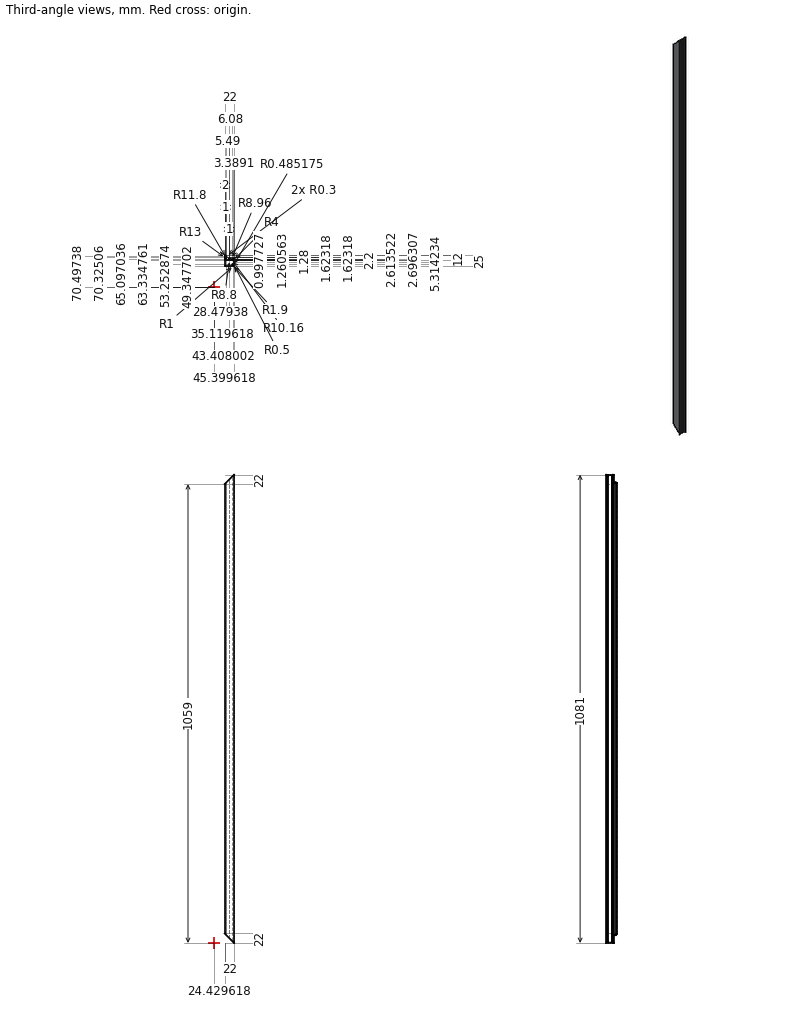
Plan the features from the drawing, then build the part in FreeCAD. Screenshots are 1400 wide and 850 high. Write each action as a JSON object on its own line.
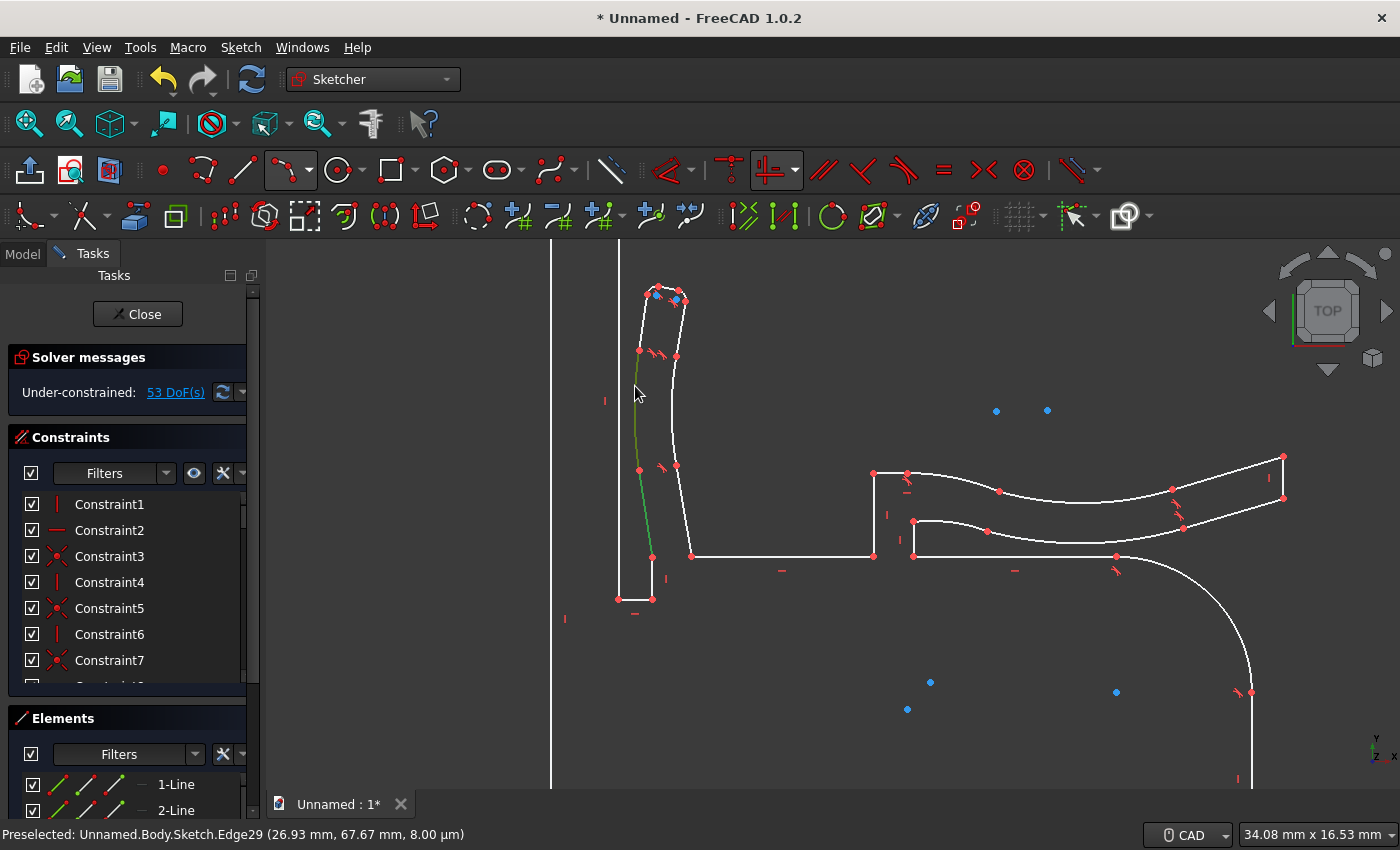
{"action": "left_click", "coordinate": [904, 170]}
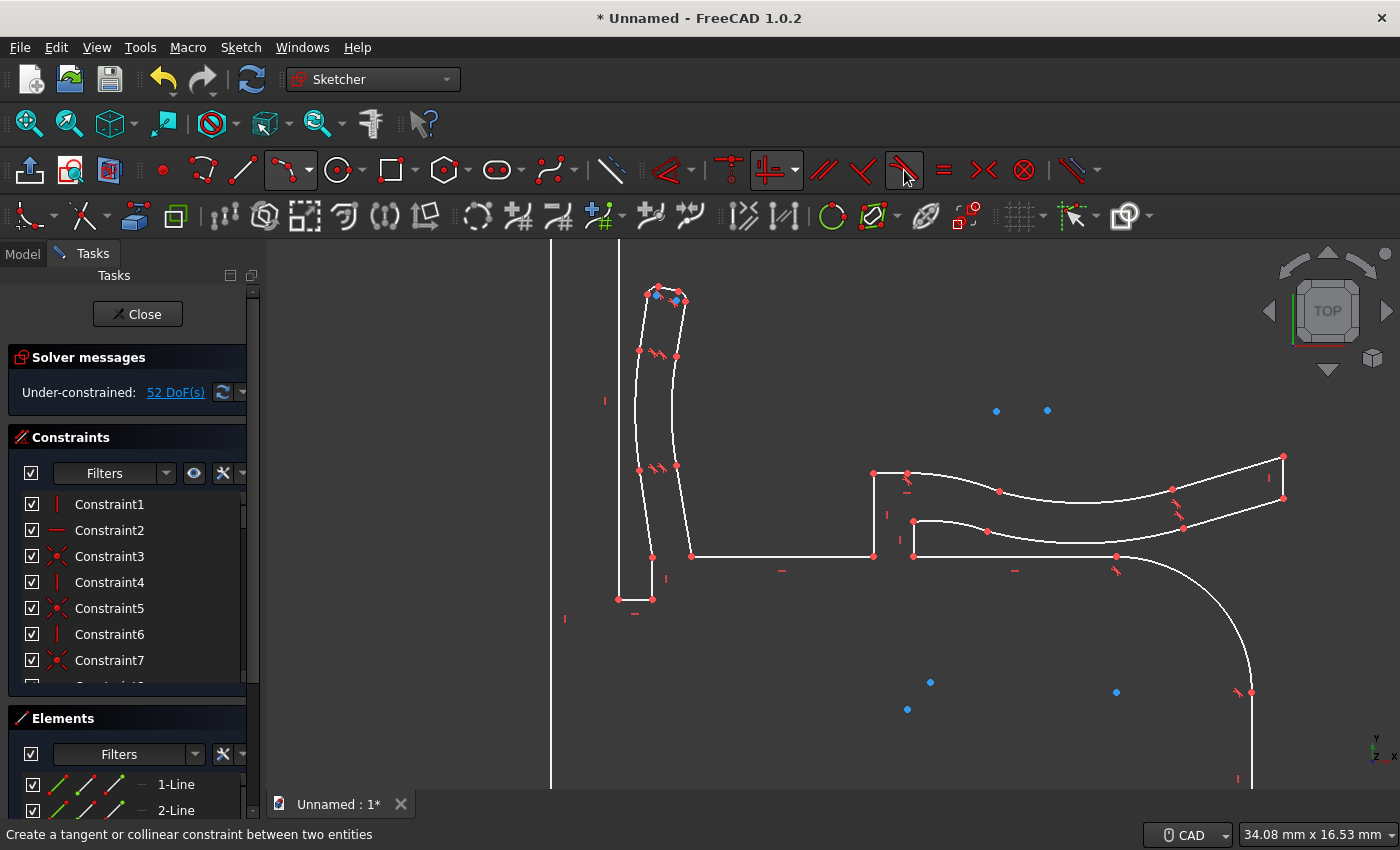
{"action": "scroll", "coordinate": [639, 431], "scroll_direction": "down", "scroll_amount": 4}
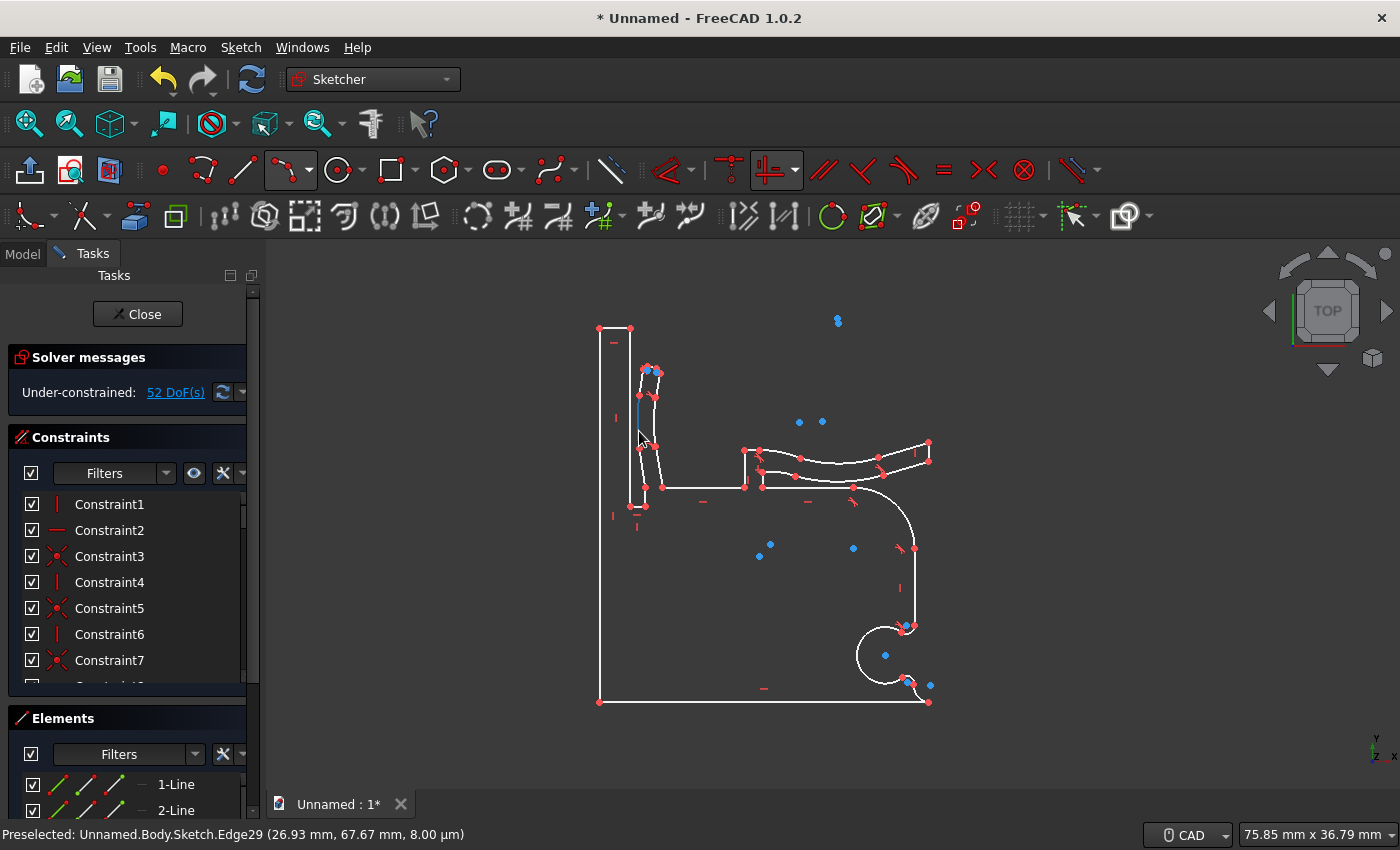
{"action": "left_click", "coordinate": [698, 702]}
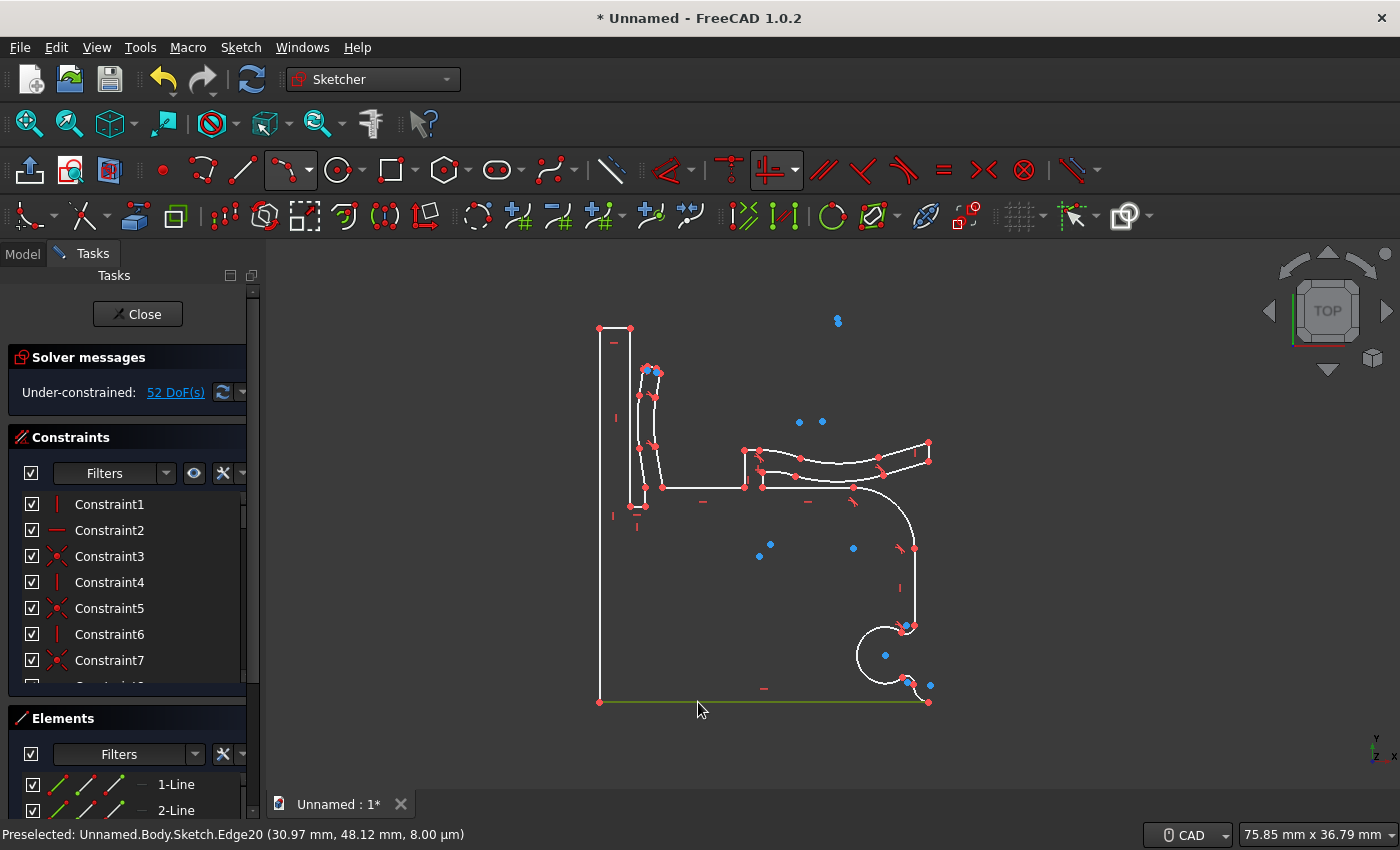
{"action": "scroll", "coordinate": [915, 692], "scroll_direction": "up", "scroll_amount": 3}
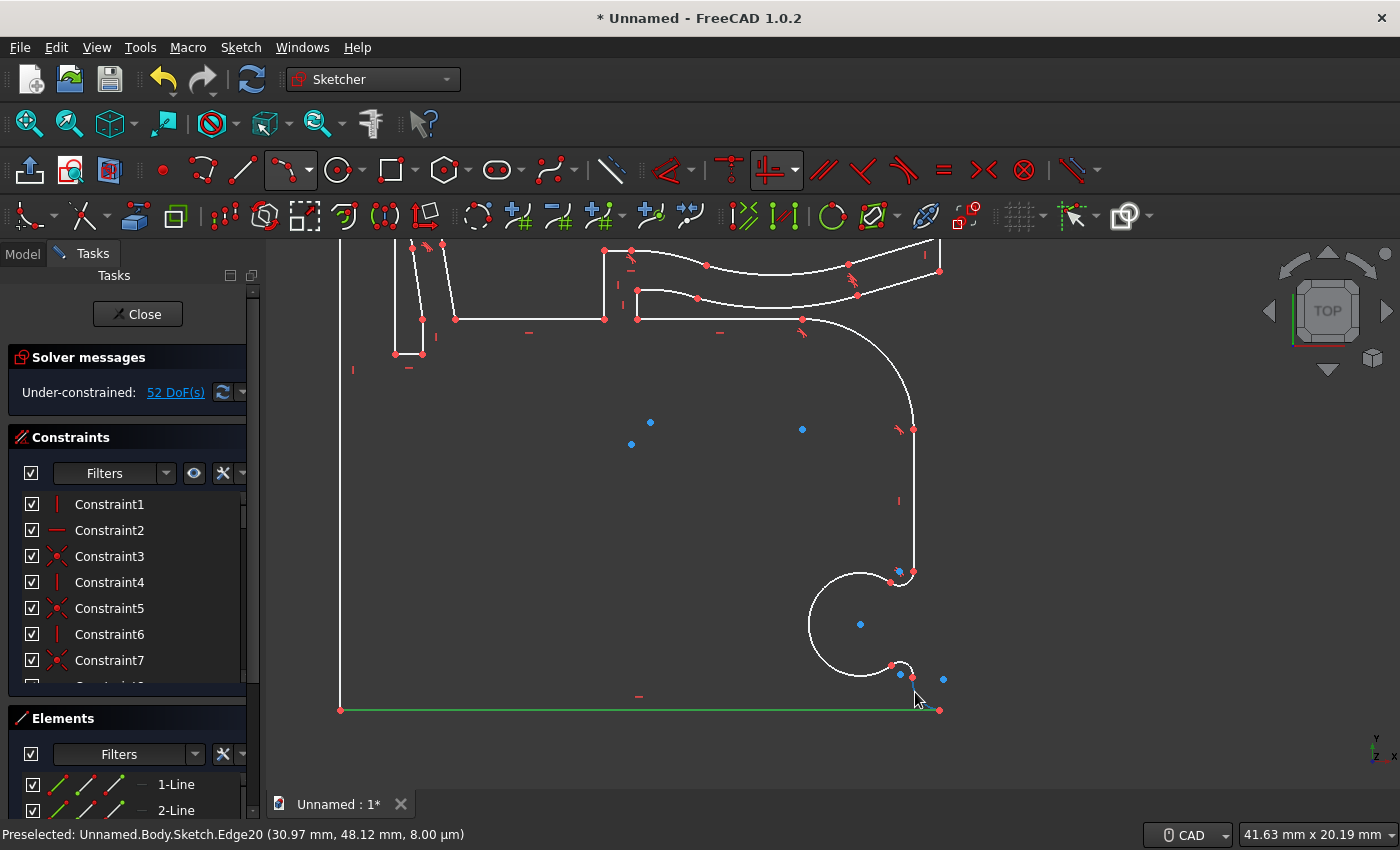
{"action": "left_click", "coordinate": [915, 692]}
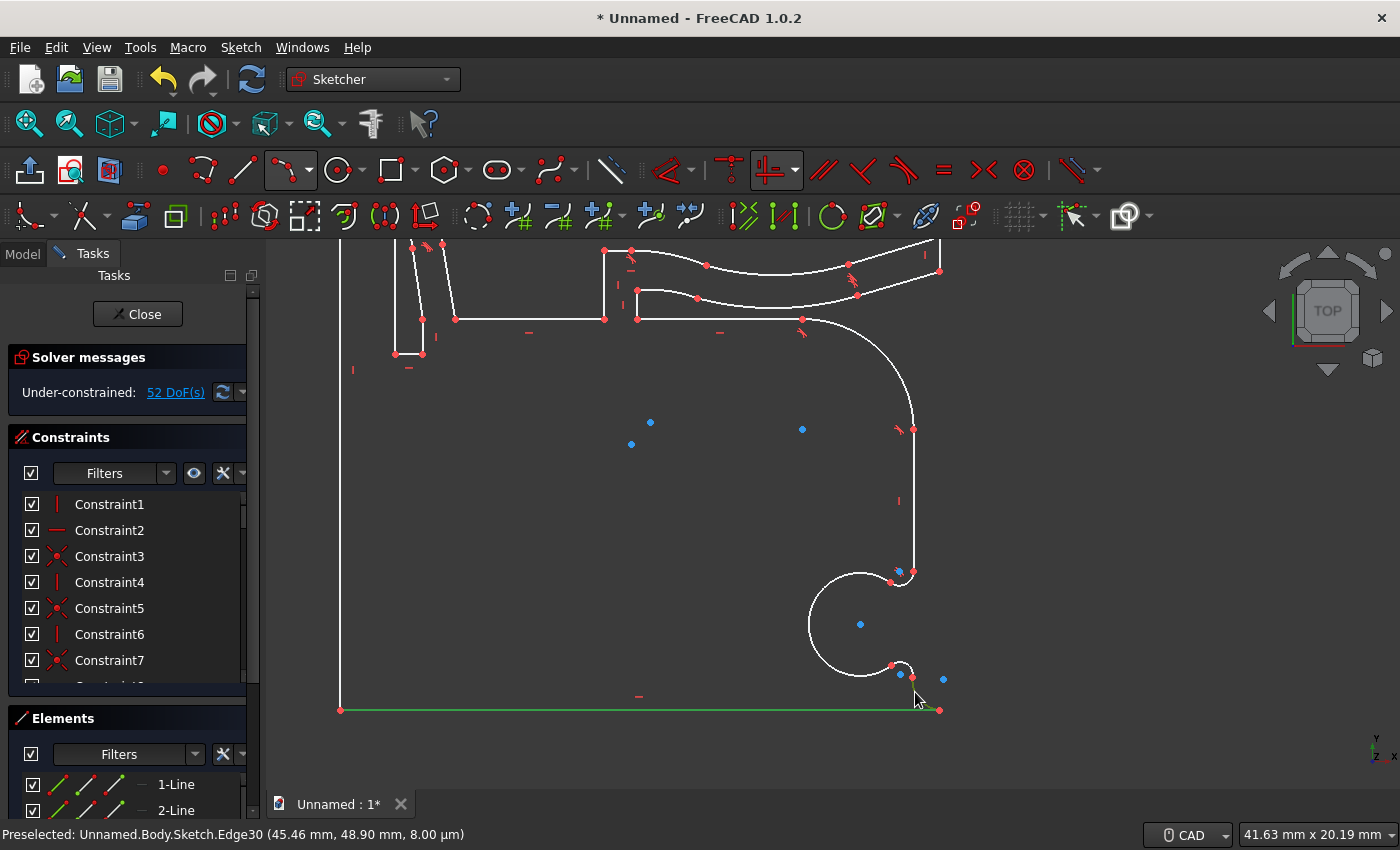
{"action": "left_click", "coordinate": [904, 170]}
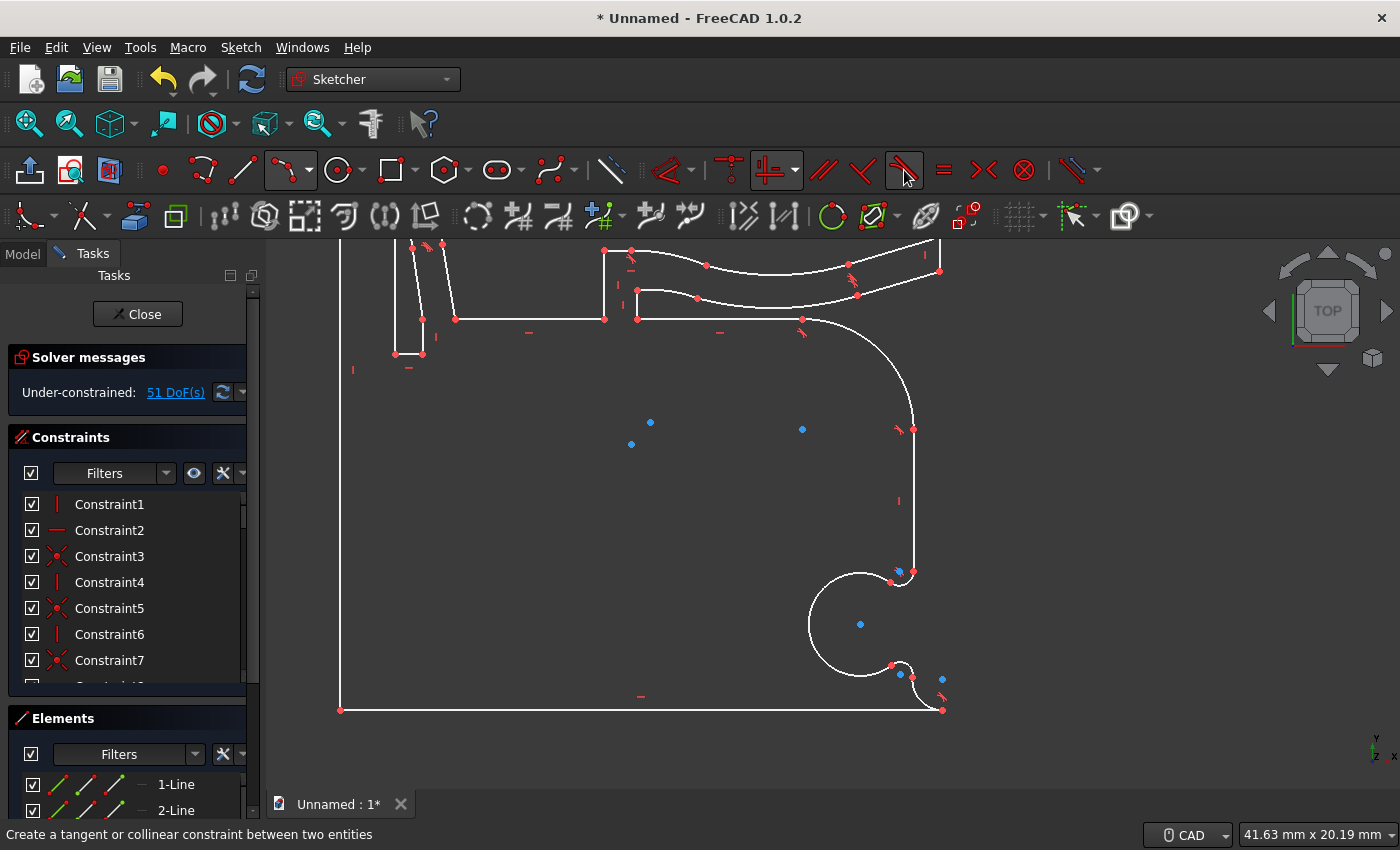
{"action": "left_click", "coordinate": [680, 293]}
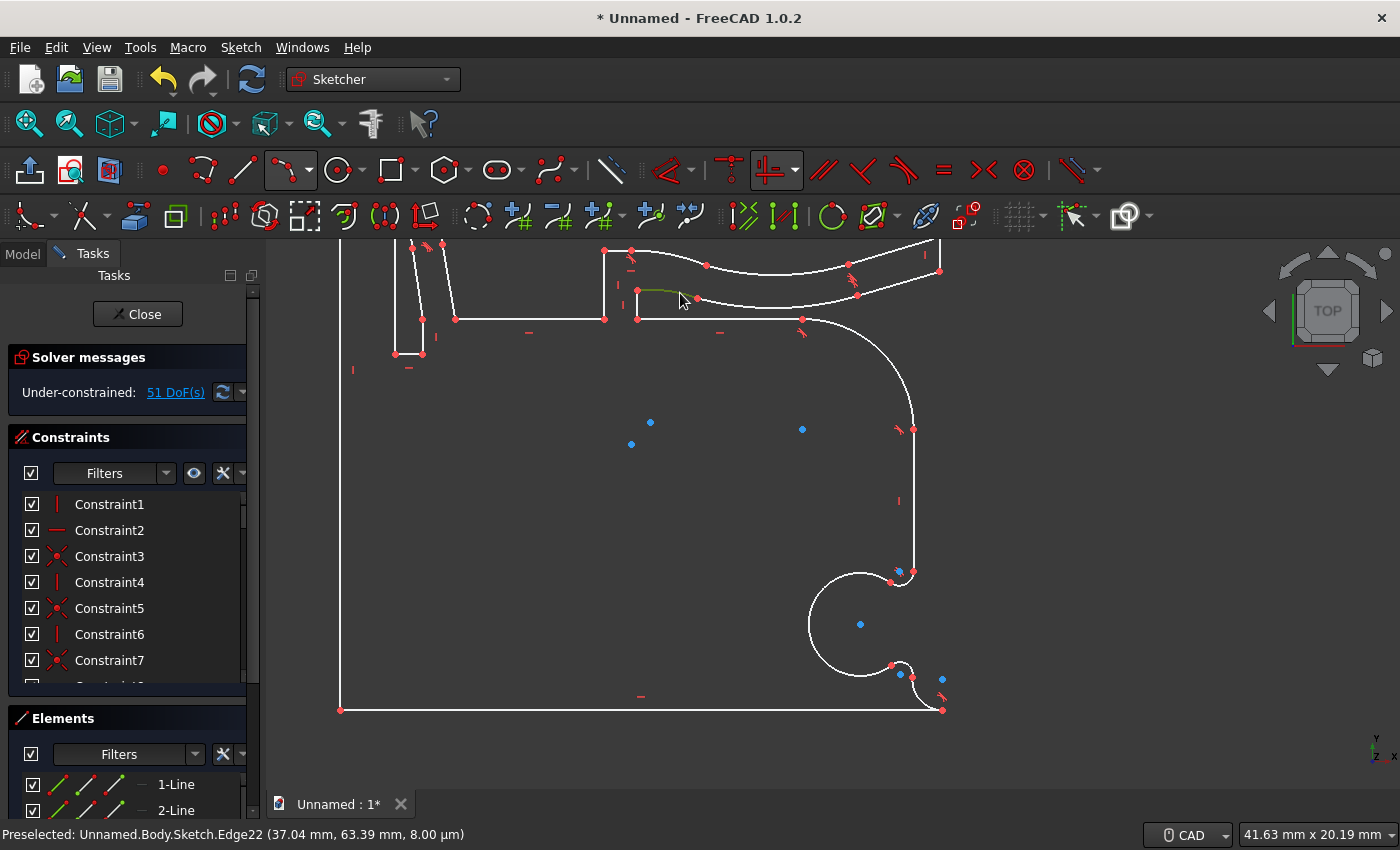
{"action": "left_click", "coordinate": [745, 307]}